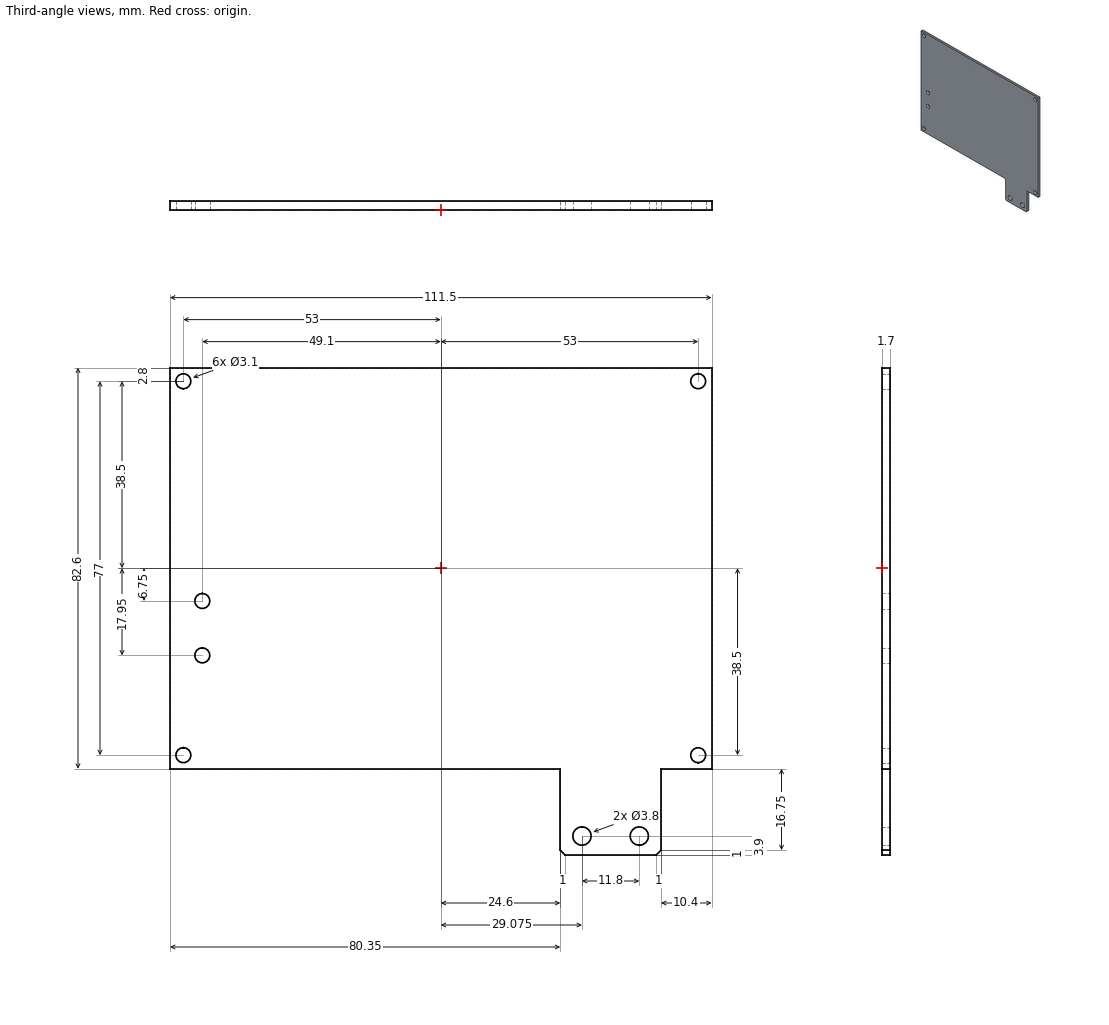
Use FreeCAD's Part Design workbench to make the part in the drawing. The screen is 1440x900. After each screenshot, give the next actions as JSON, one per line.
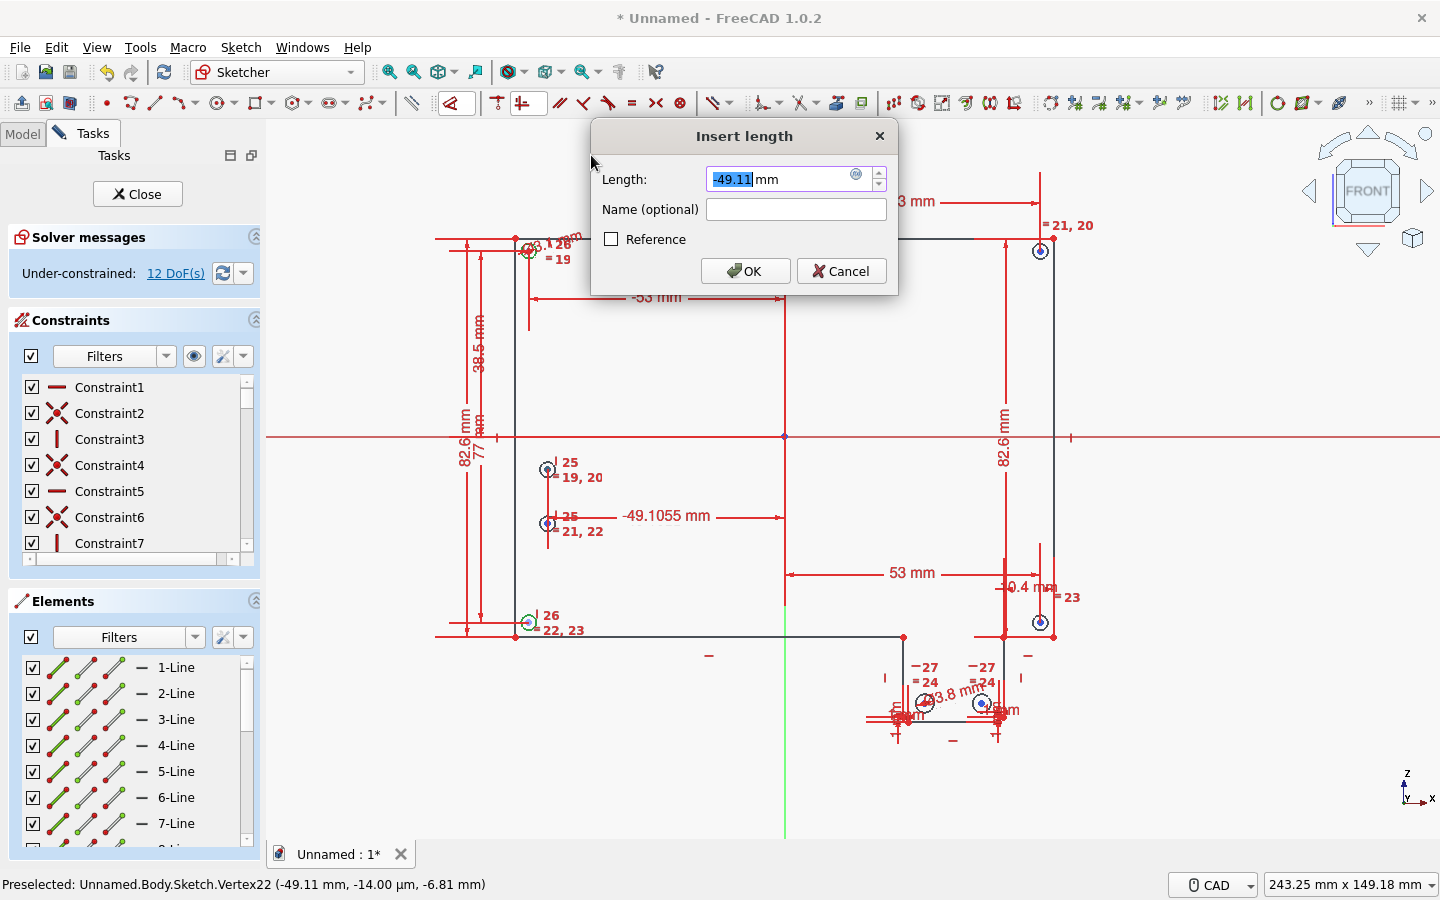
{"action": "type", "text": "-49.1"}
{"action": "key", "text": "Return"}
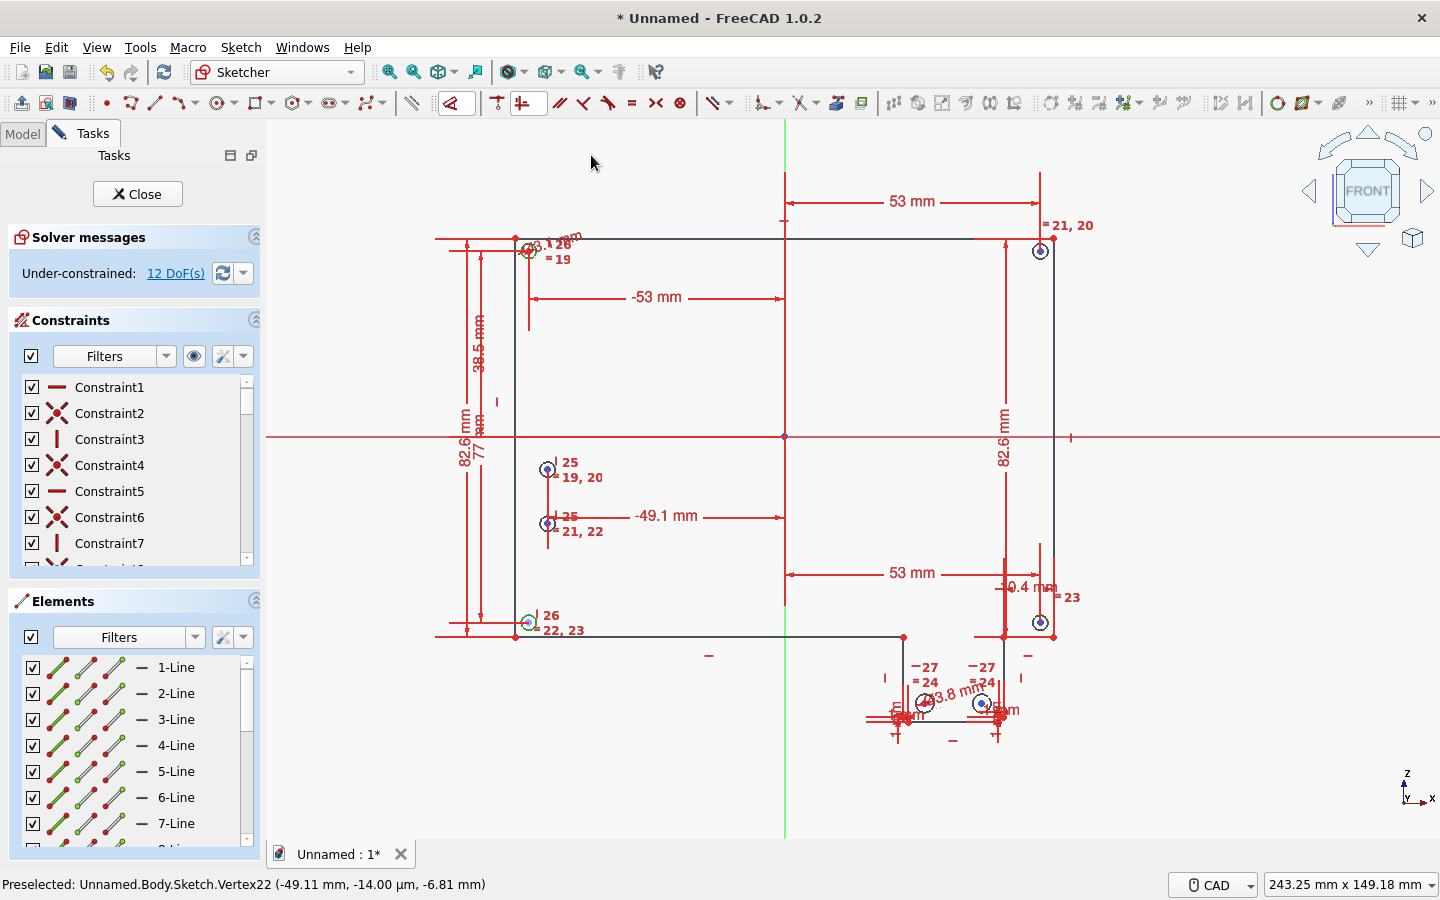
{"action": "left_click", "coordinate": [548, 470]}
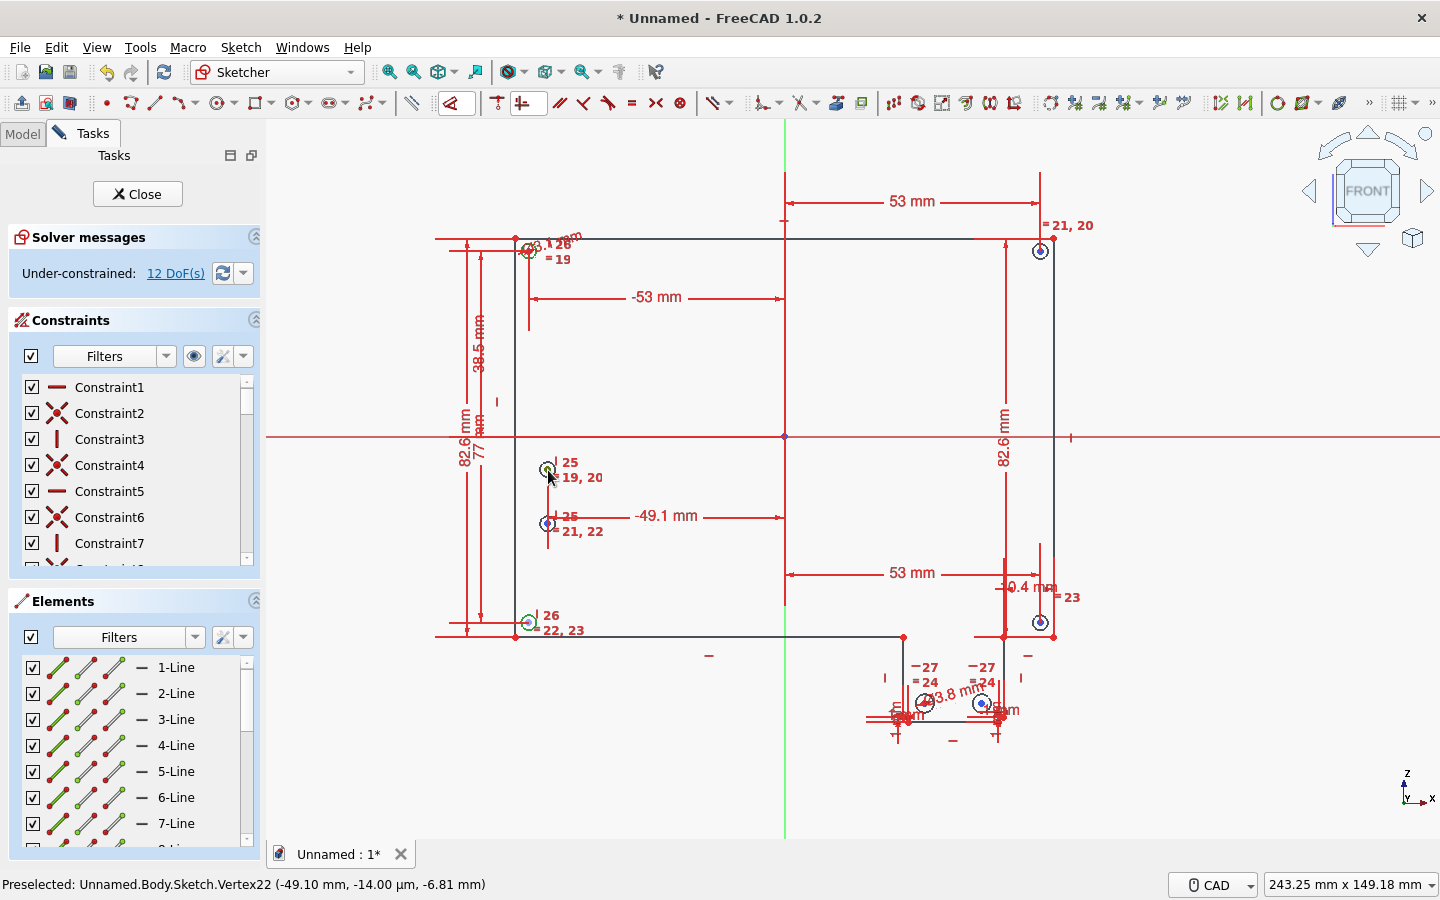
{"action": "left_click", "coordinate": [470, 104]}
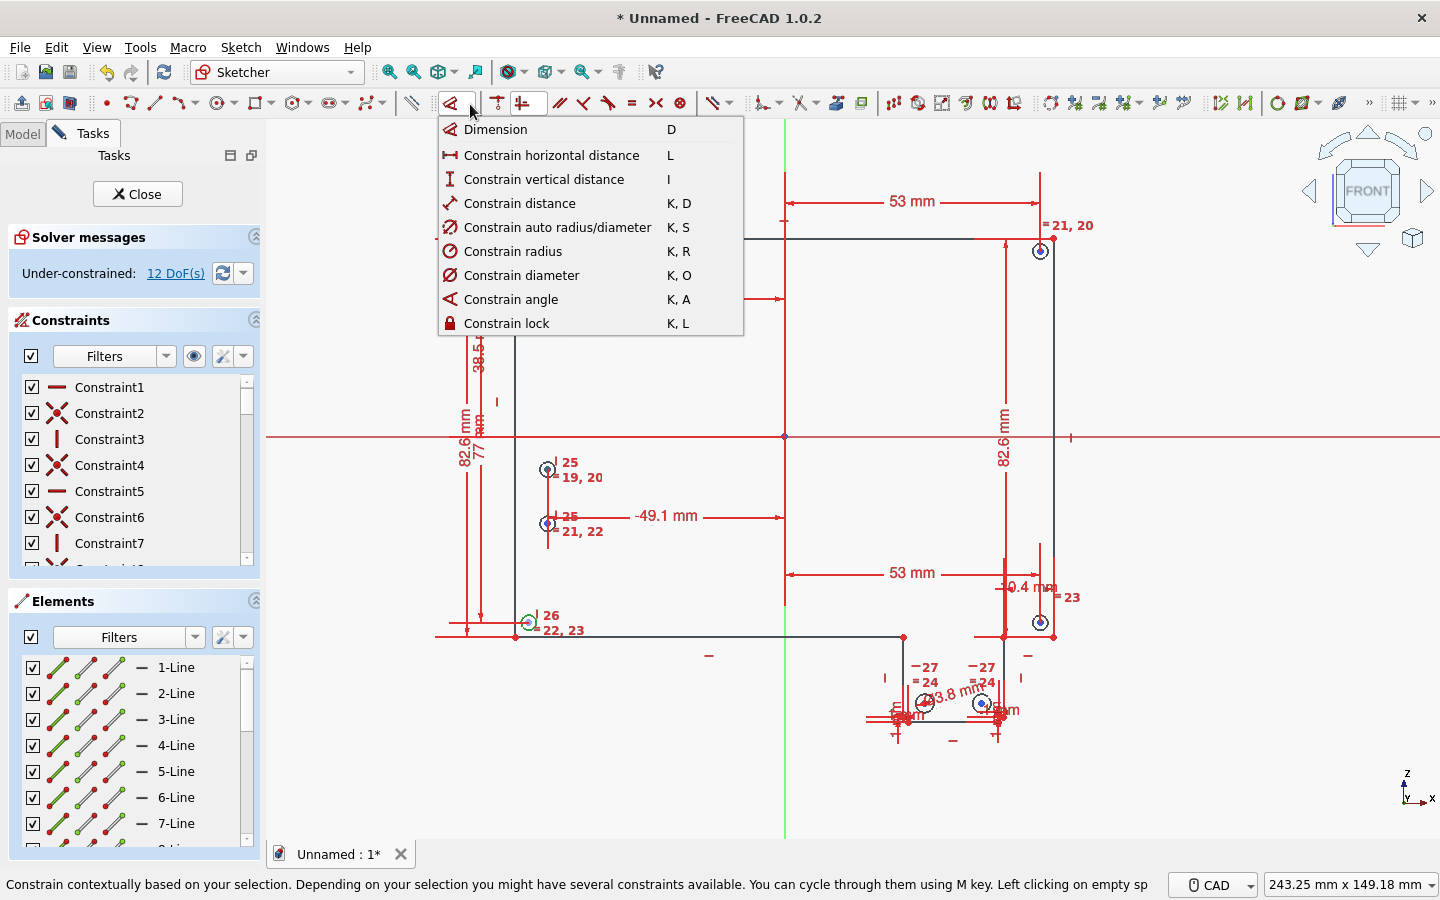
{"action": "left_click", "coordinate": [591, 179]}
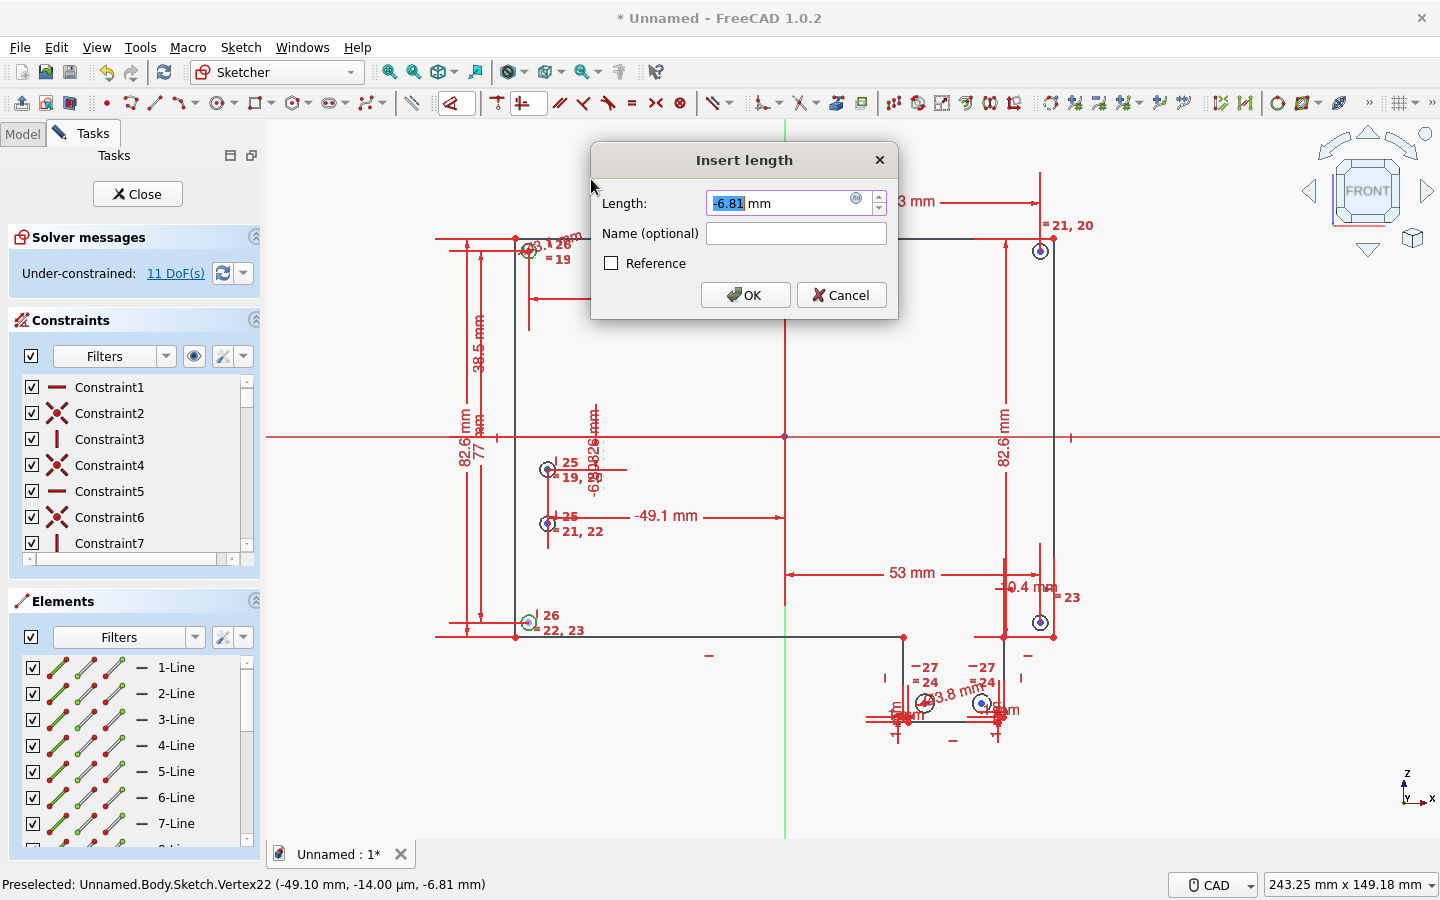
{"action": "type", "text": "-6.75"}
{"action": "key", "text": "Return"}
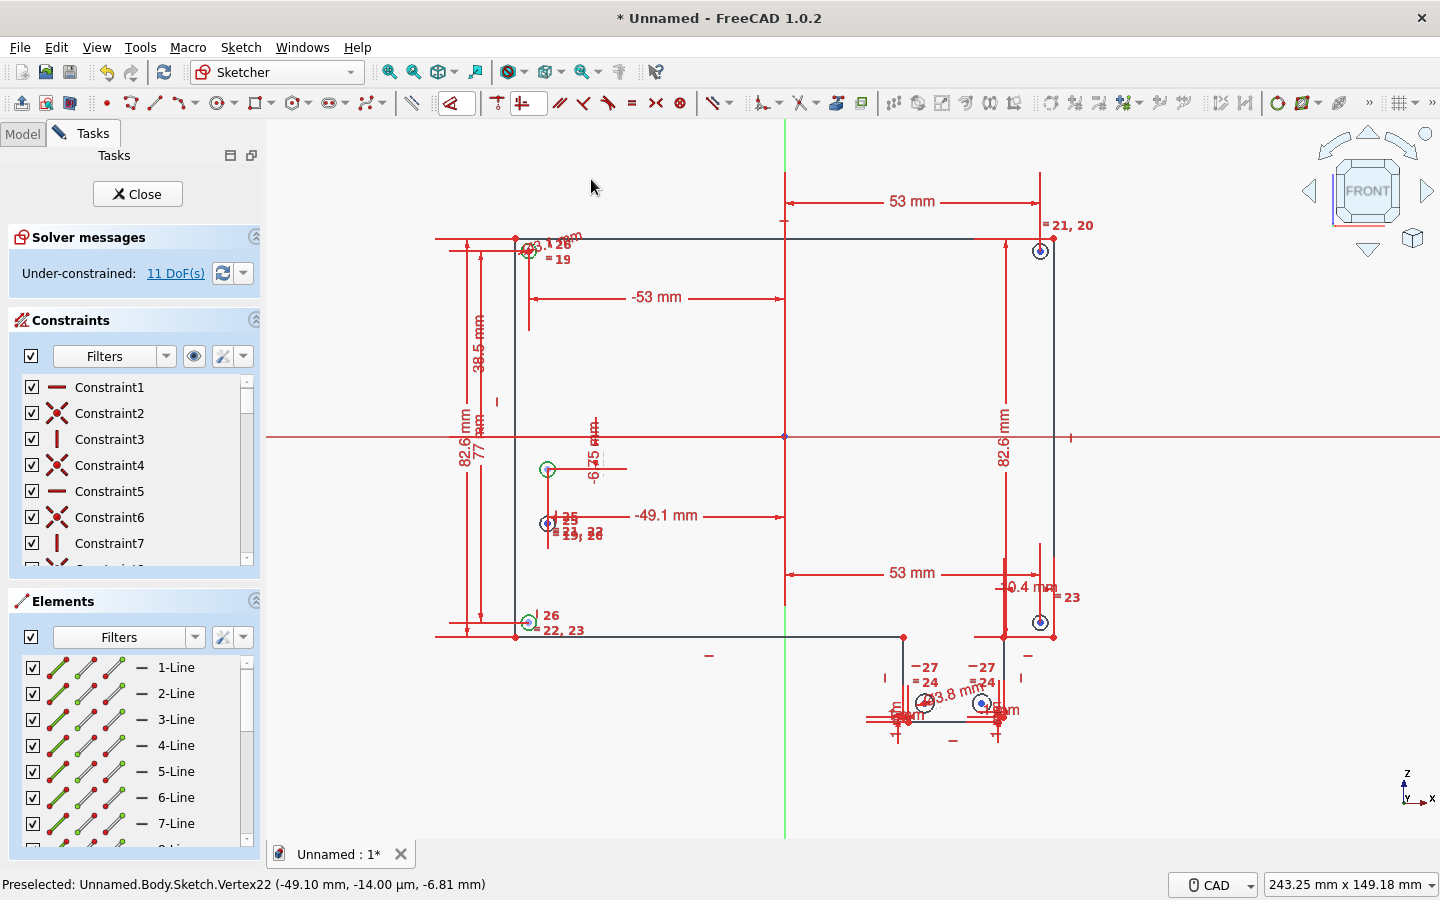
{"action": "left_click", "coordinate": [1040, 251]}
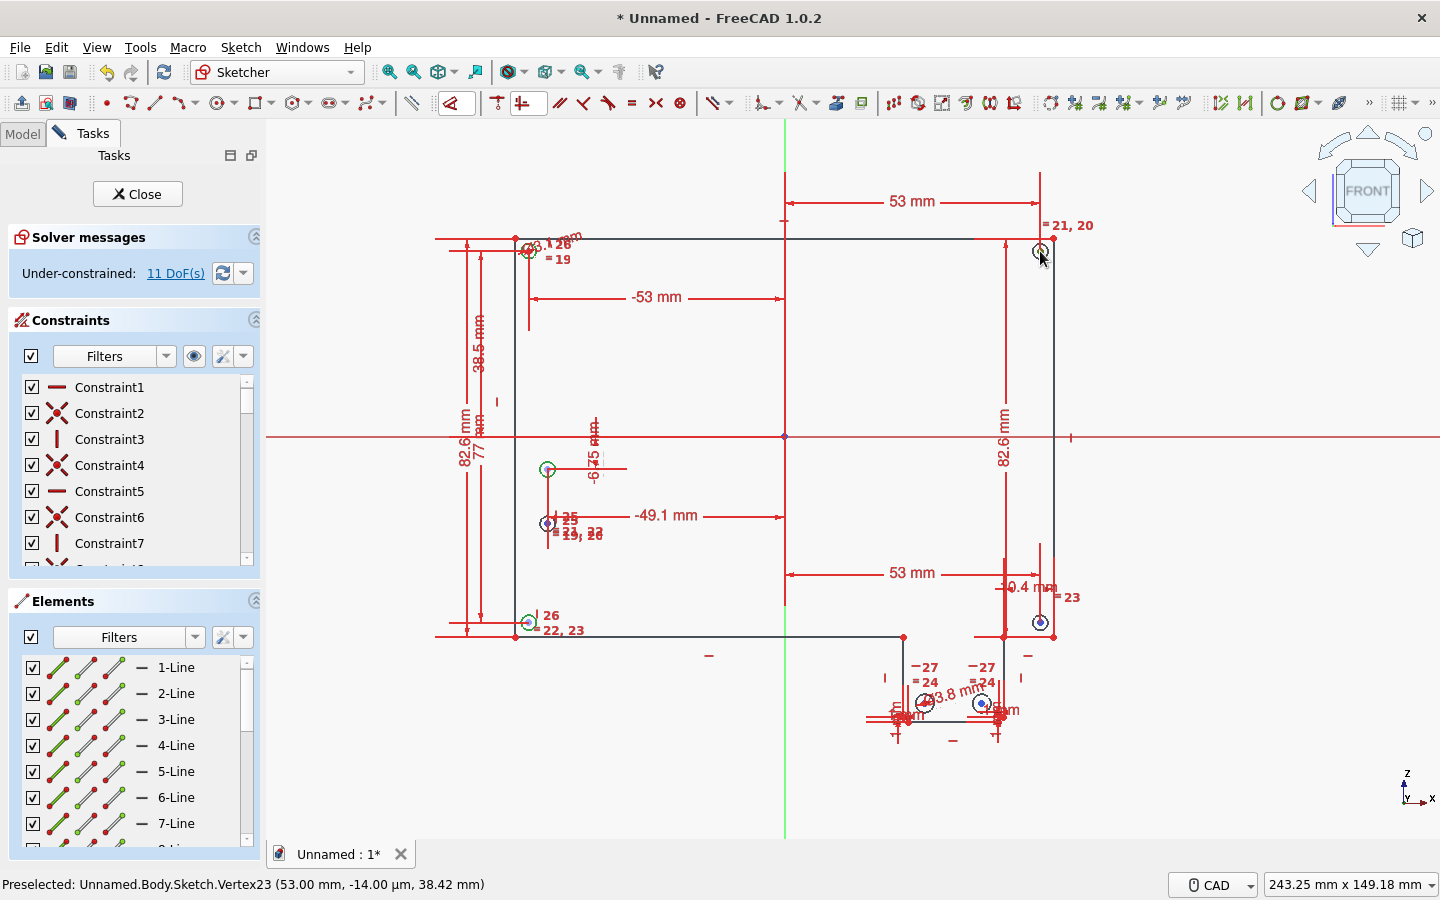
{"action": "key", "text": "i"}